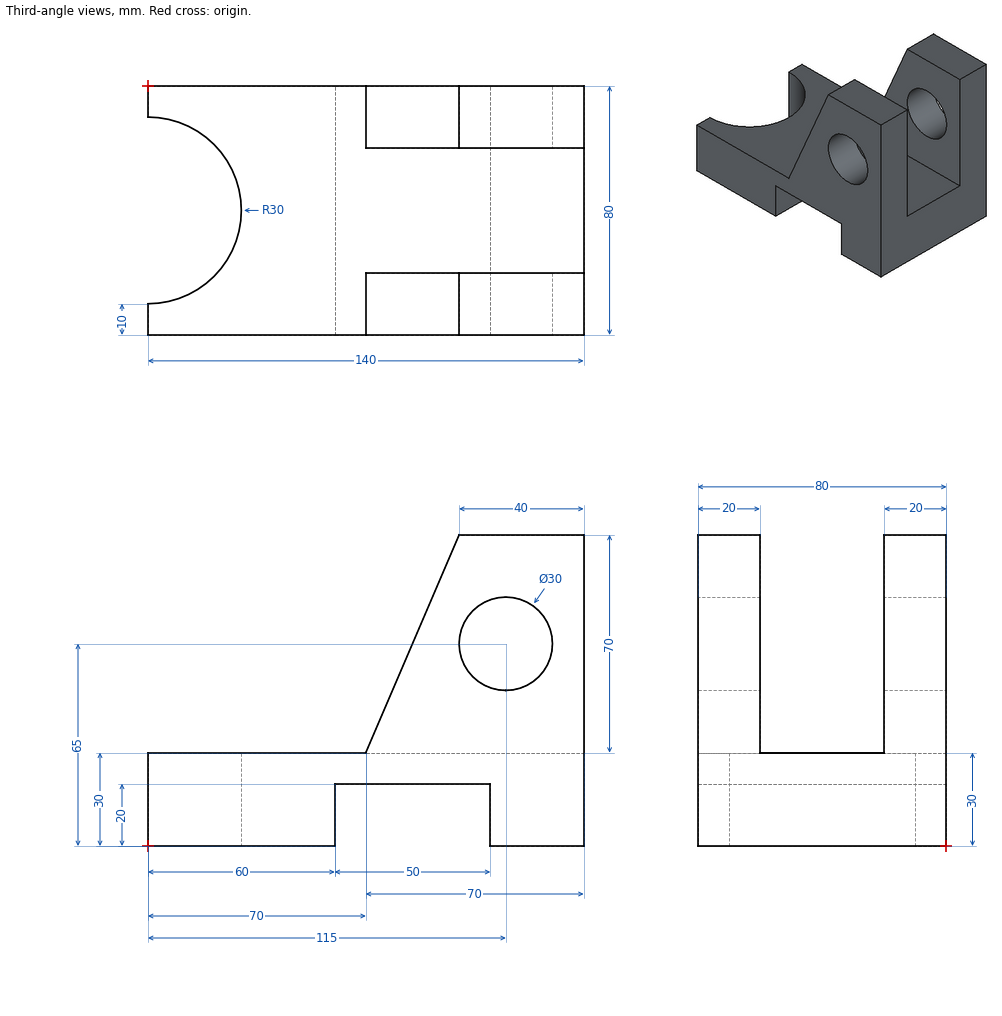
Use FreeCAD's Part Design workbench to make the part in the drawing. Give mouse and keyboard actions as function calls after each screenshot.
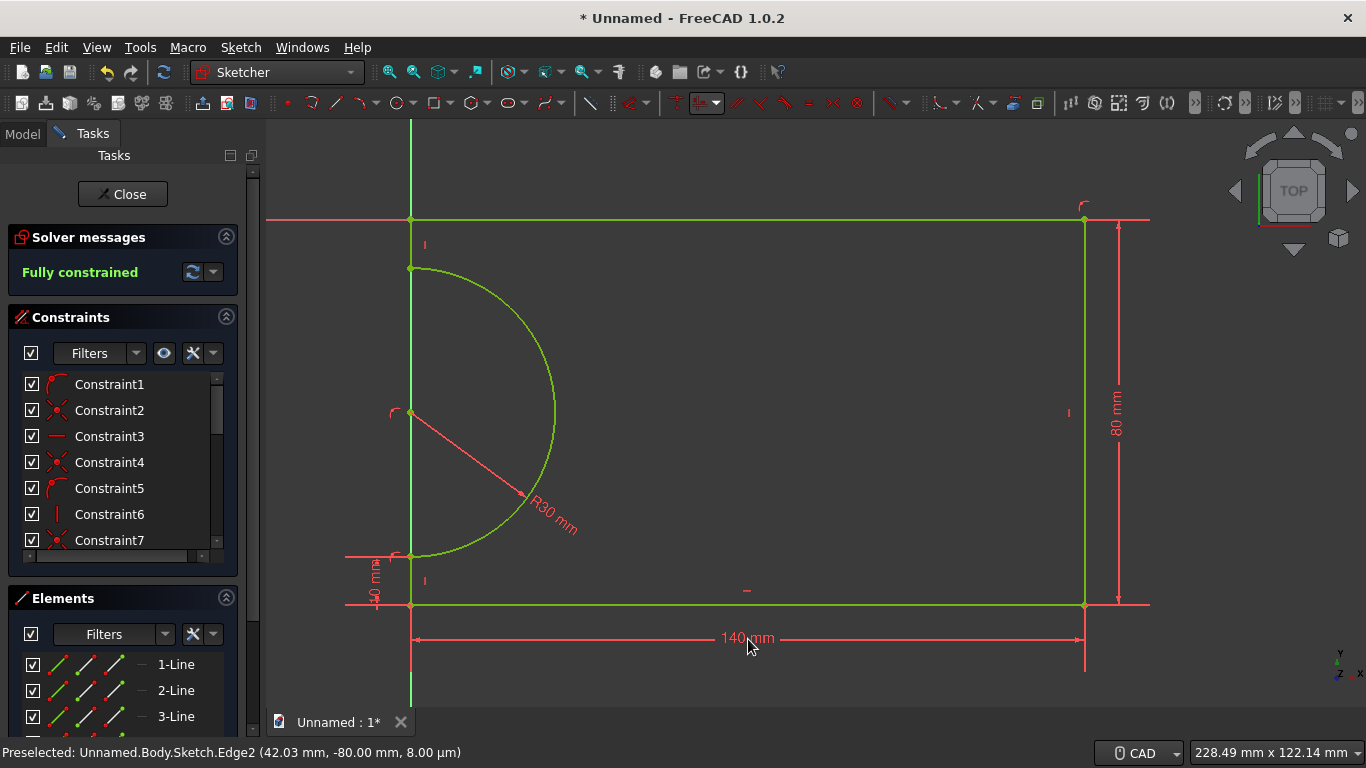
click(123, 194)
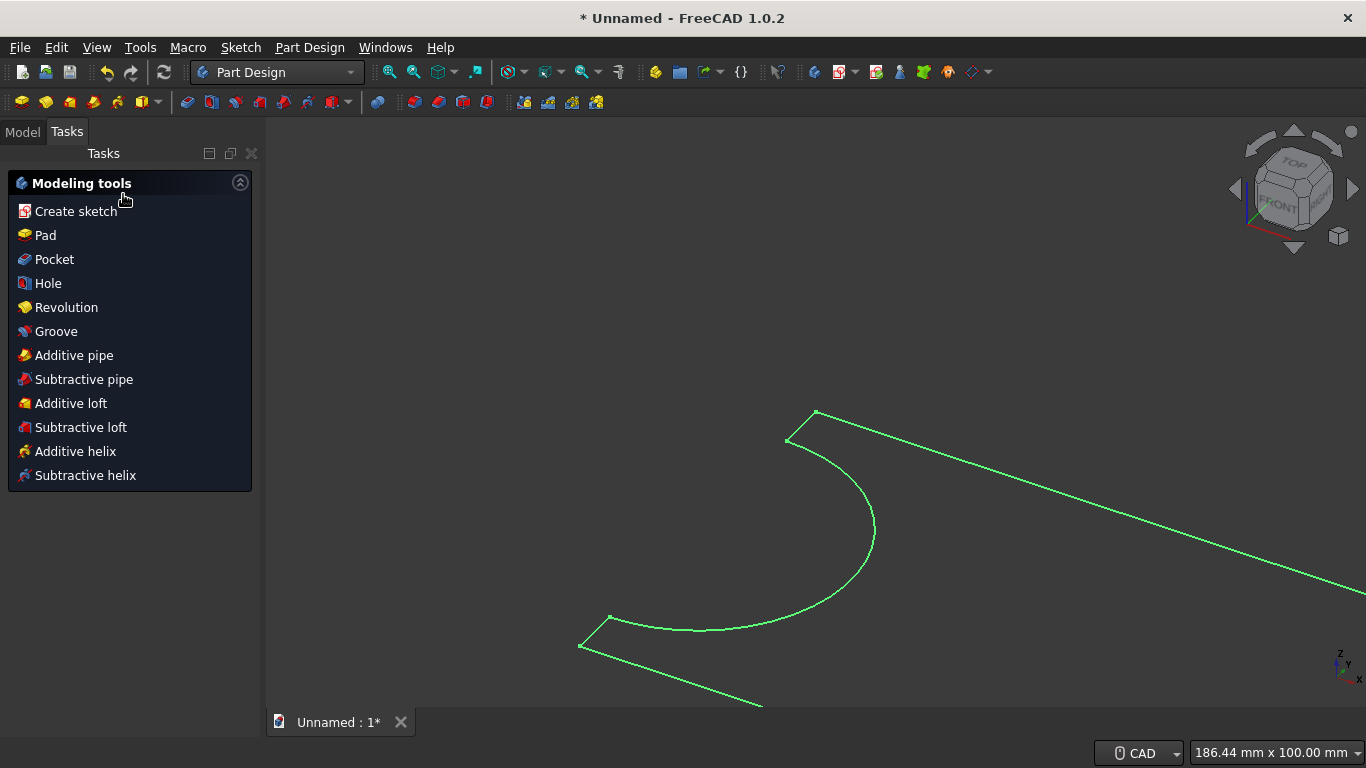
click(22, 102)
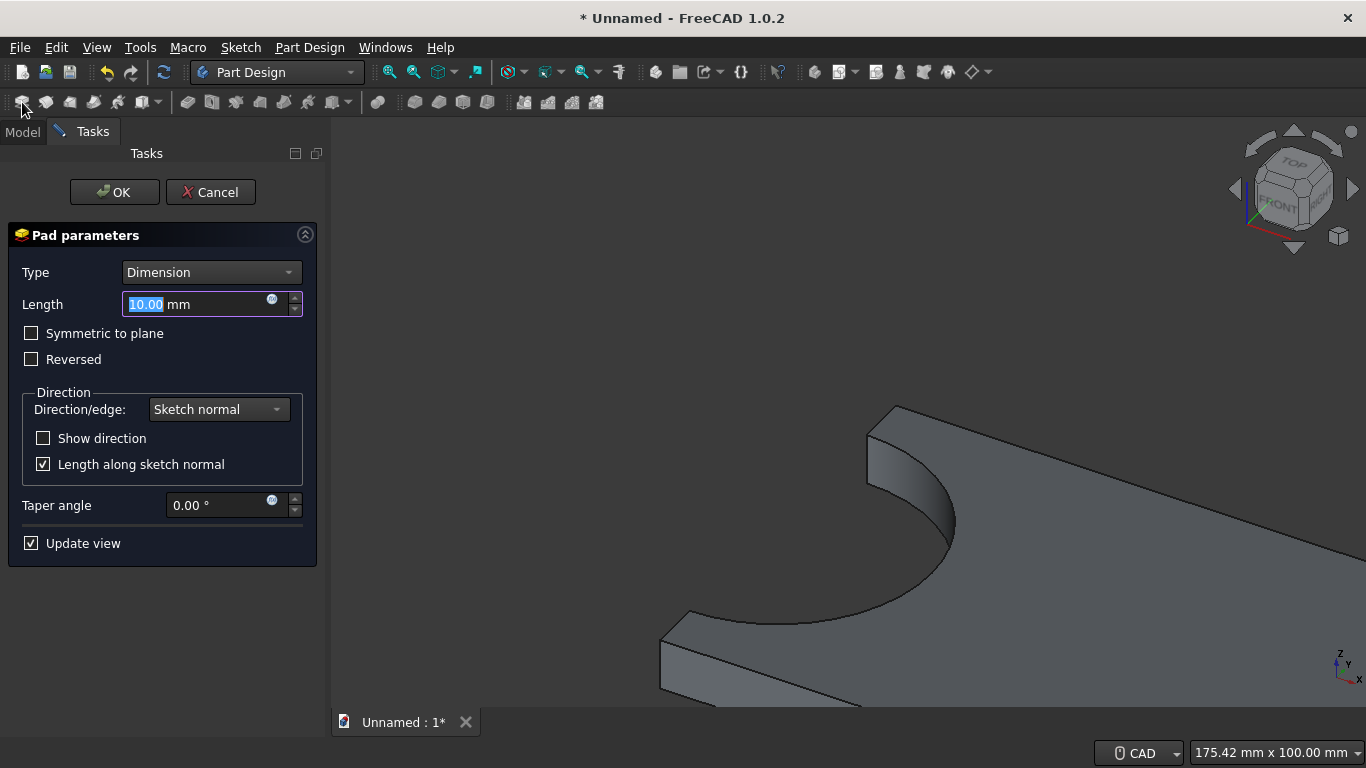
text(30)
key(Tab)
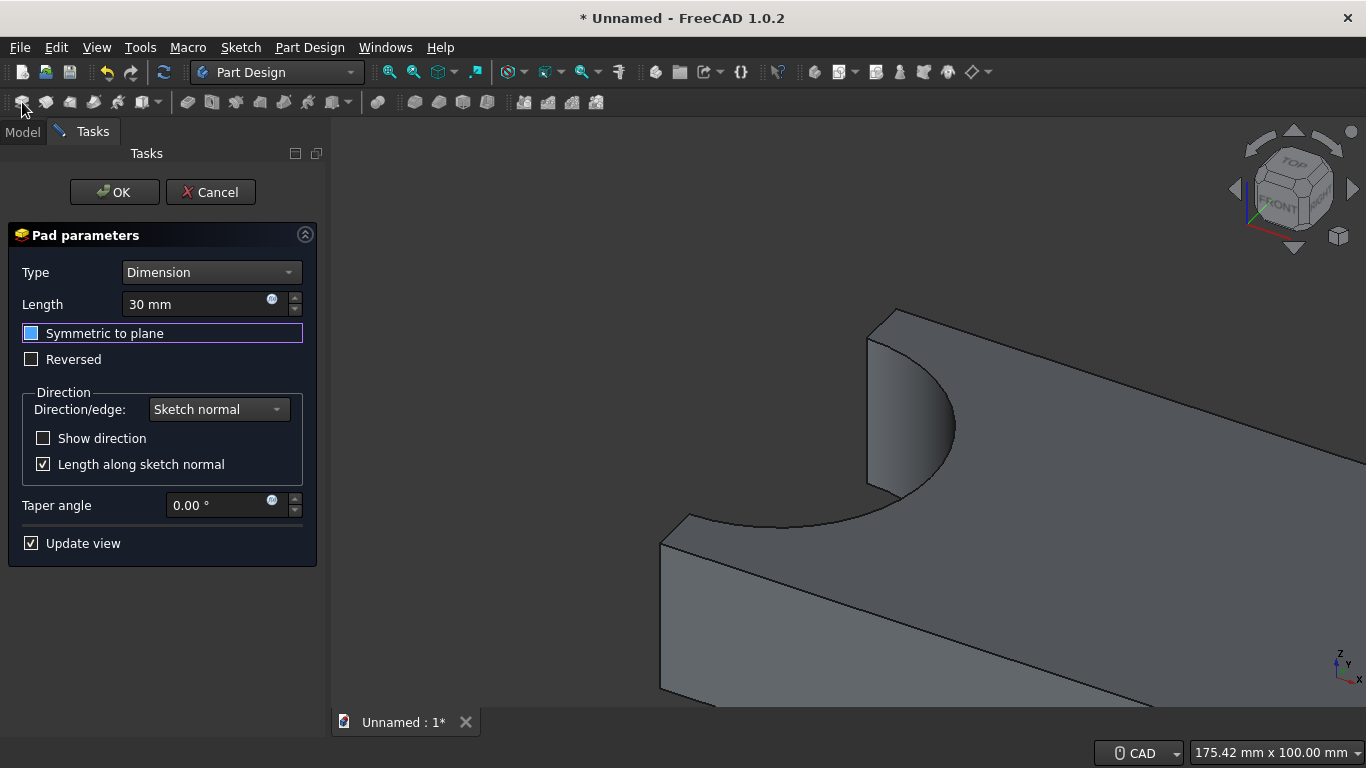
click(115, 192)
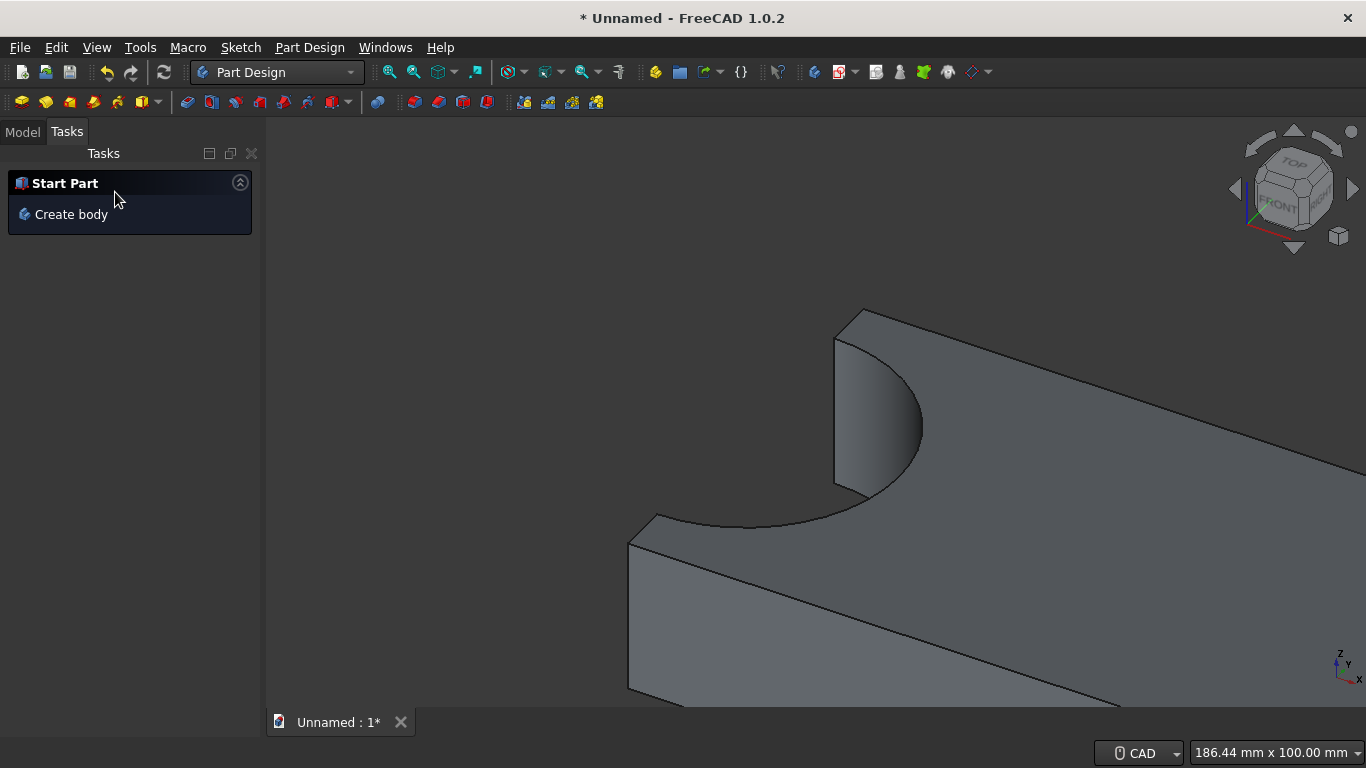
click(390, 72)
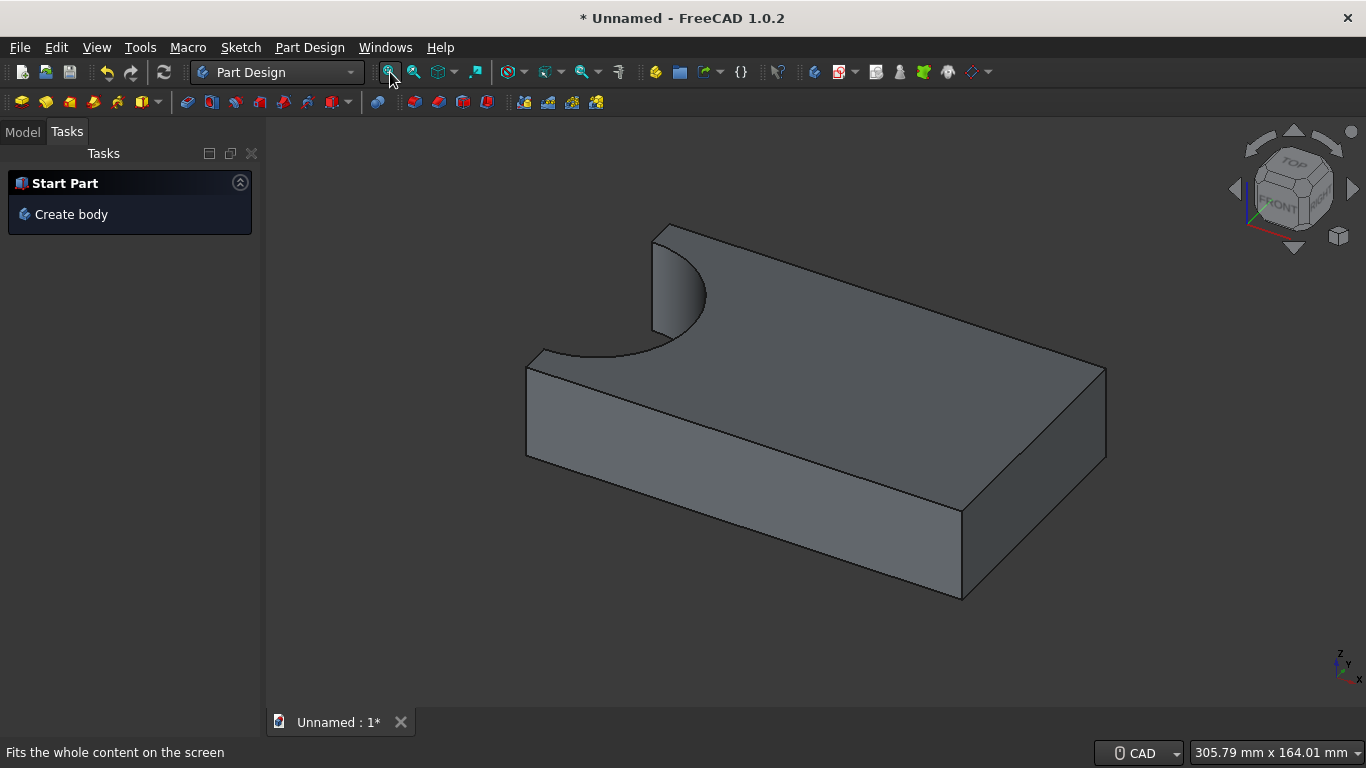
click(869, 524)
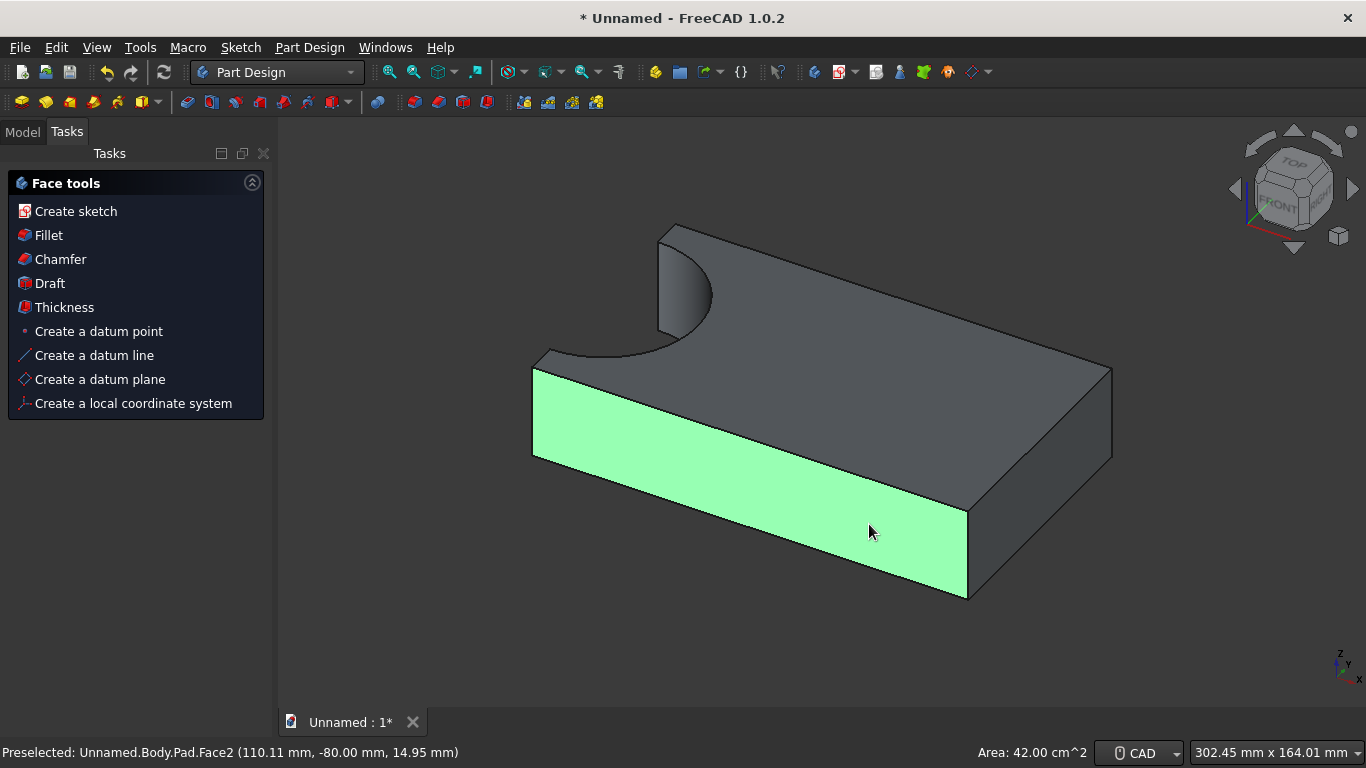
click(840, 72)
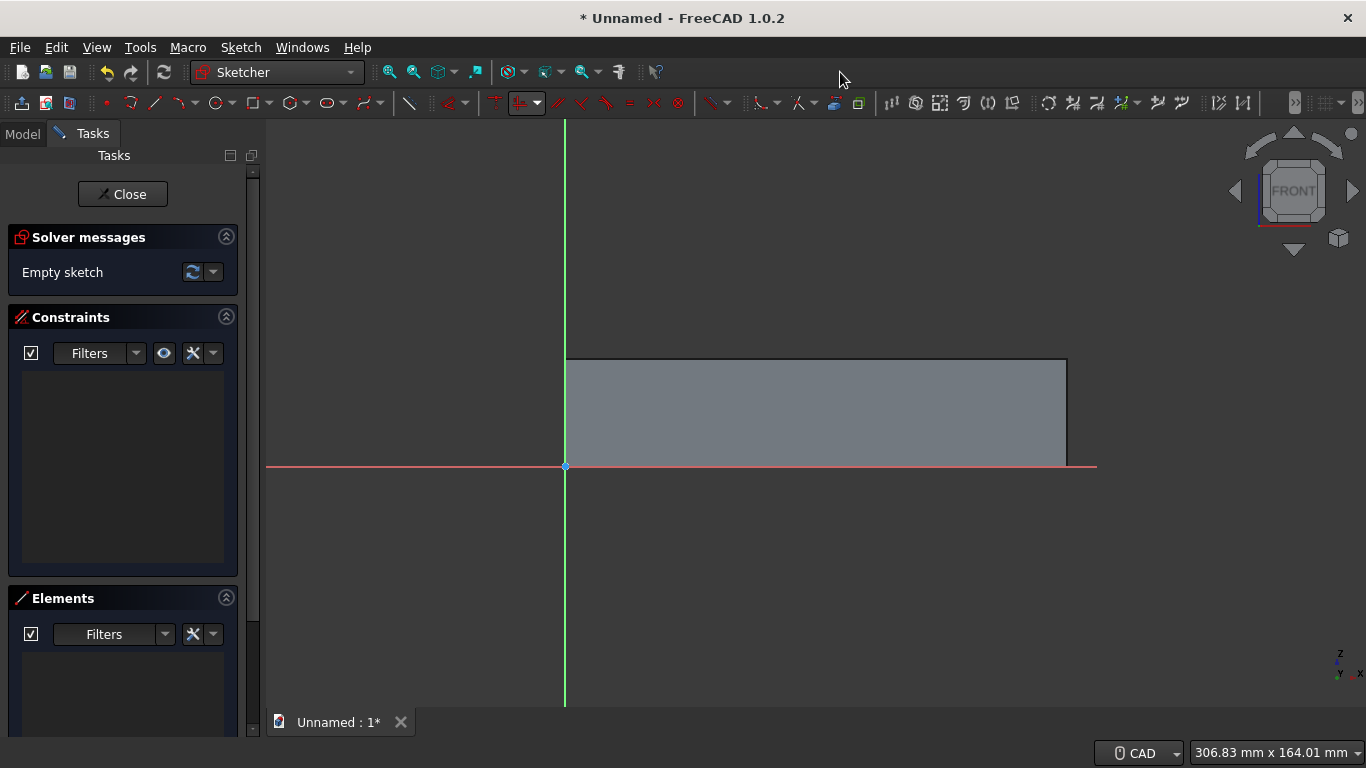
scroll(438, 679, down, 1)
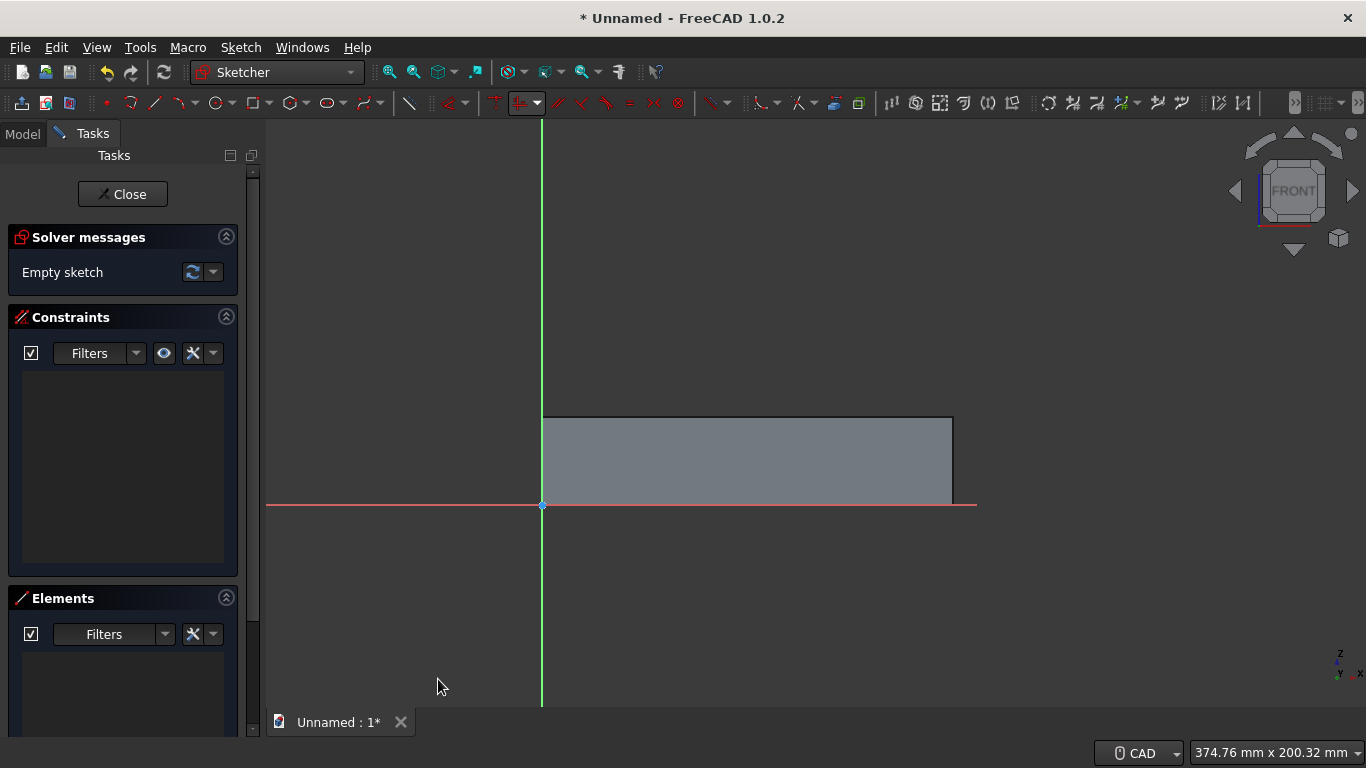
click(132, 104)